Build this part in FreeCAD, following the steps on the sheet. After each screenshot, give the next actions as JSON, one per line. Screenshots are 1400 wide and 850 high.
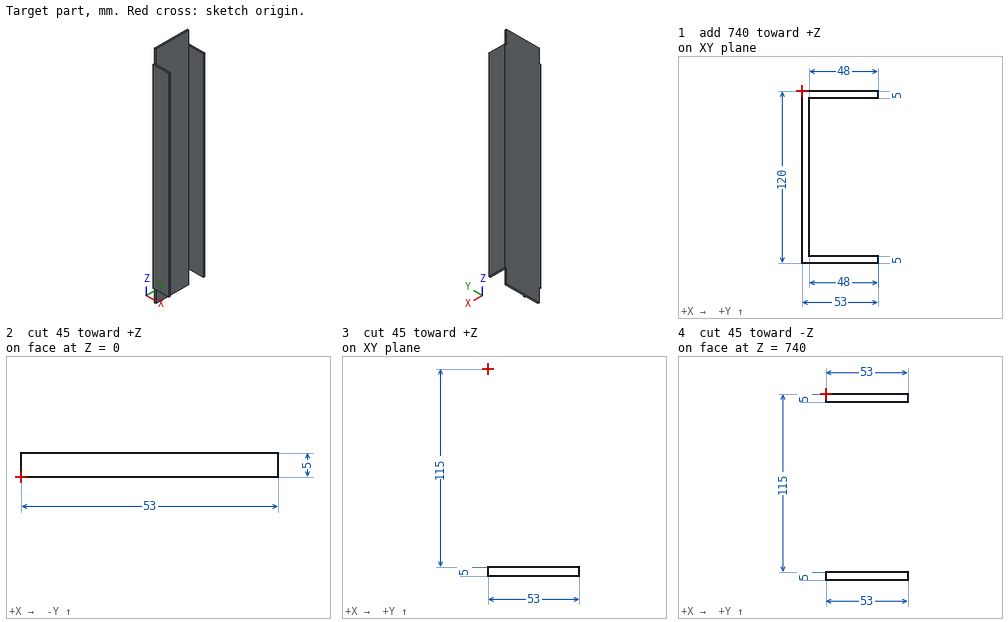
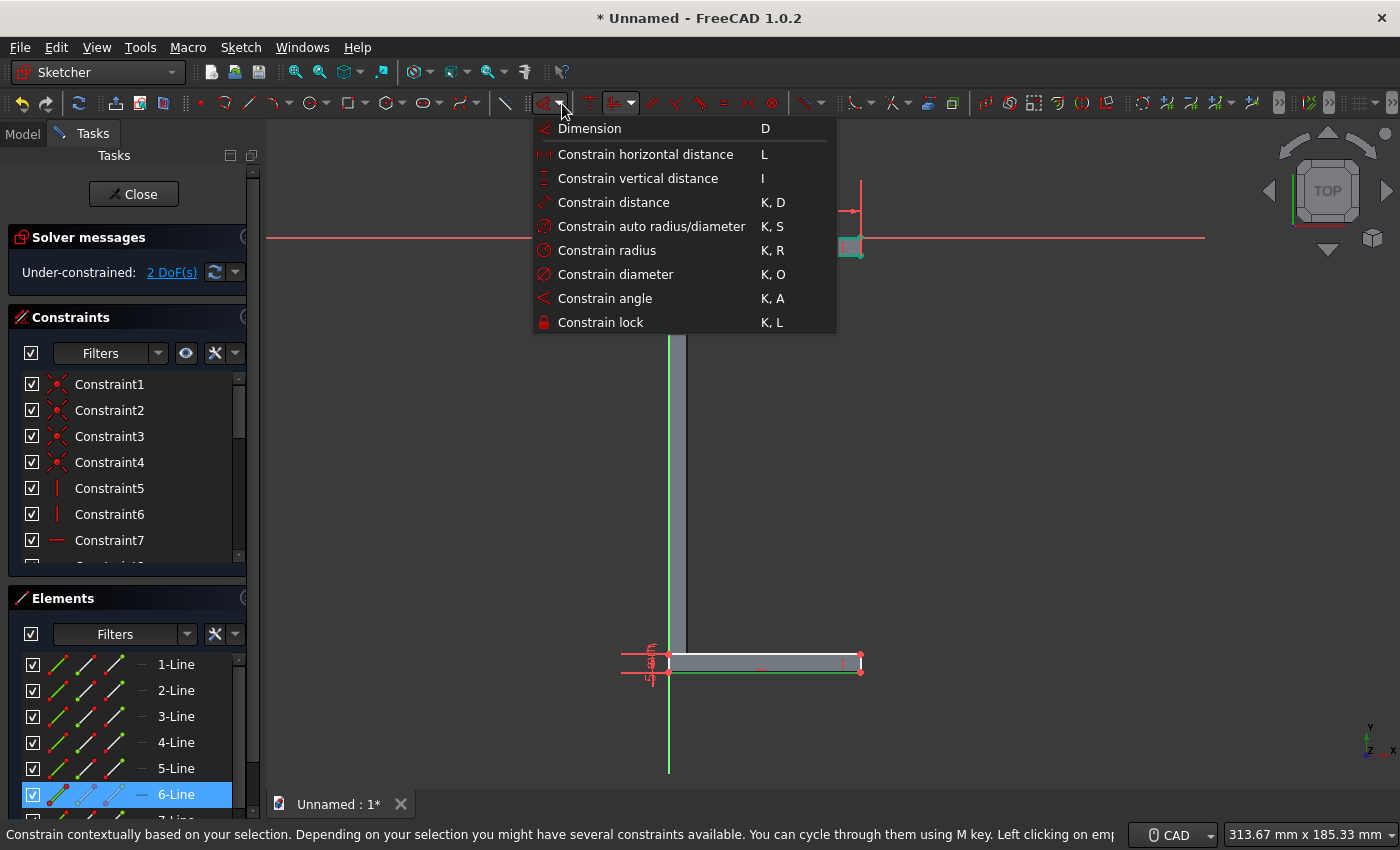
{"action": "left_click", "coordinate": [685, 154]}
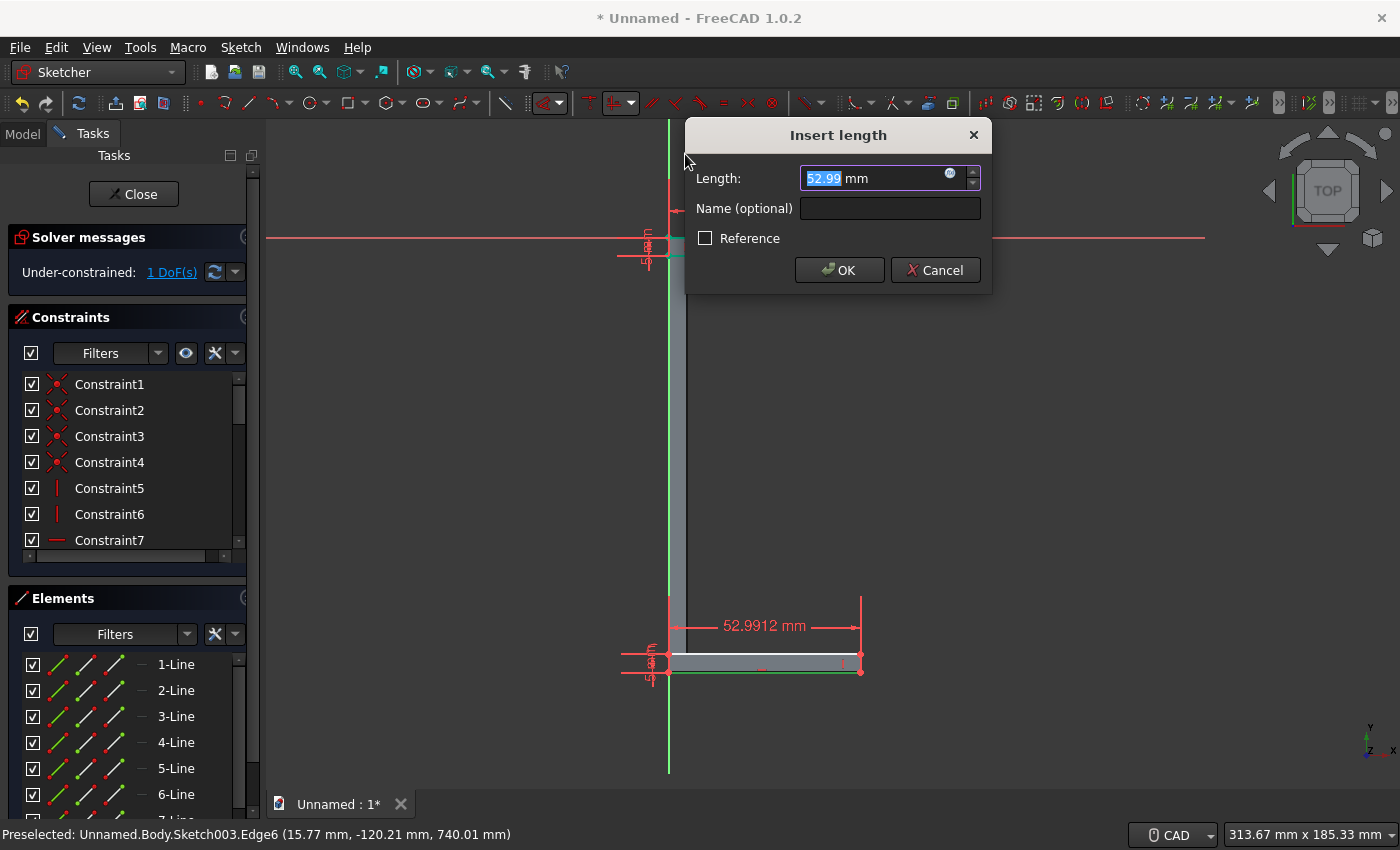
{"action": "type", "text": "53"}
{"action": "key", "text": "Return"}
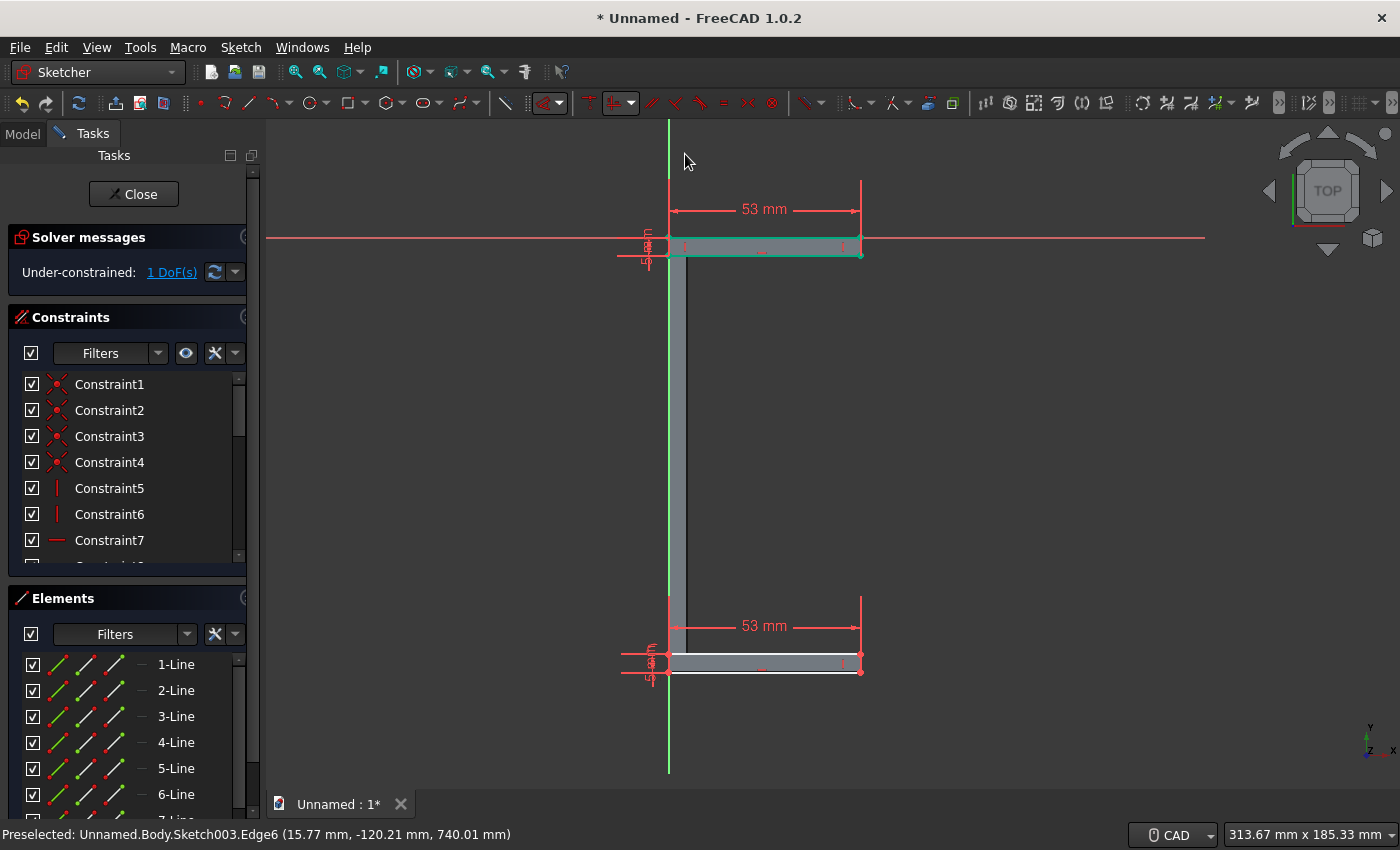
{"action": "left_click", "coordinate": [669, 654]}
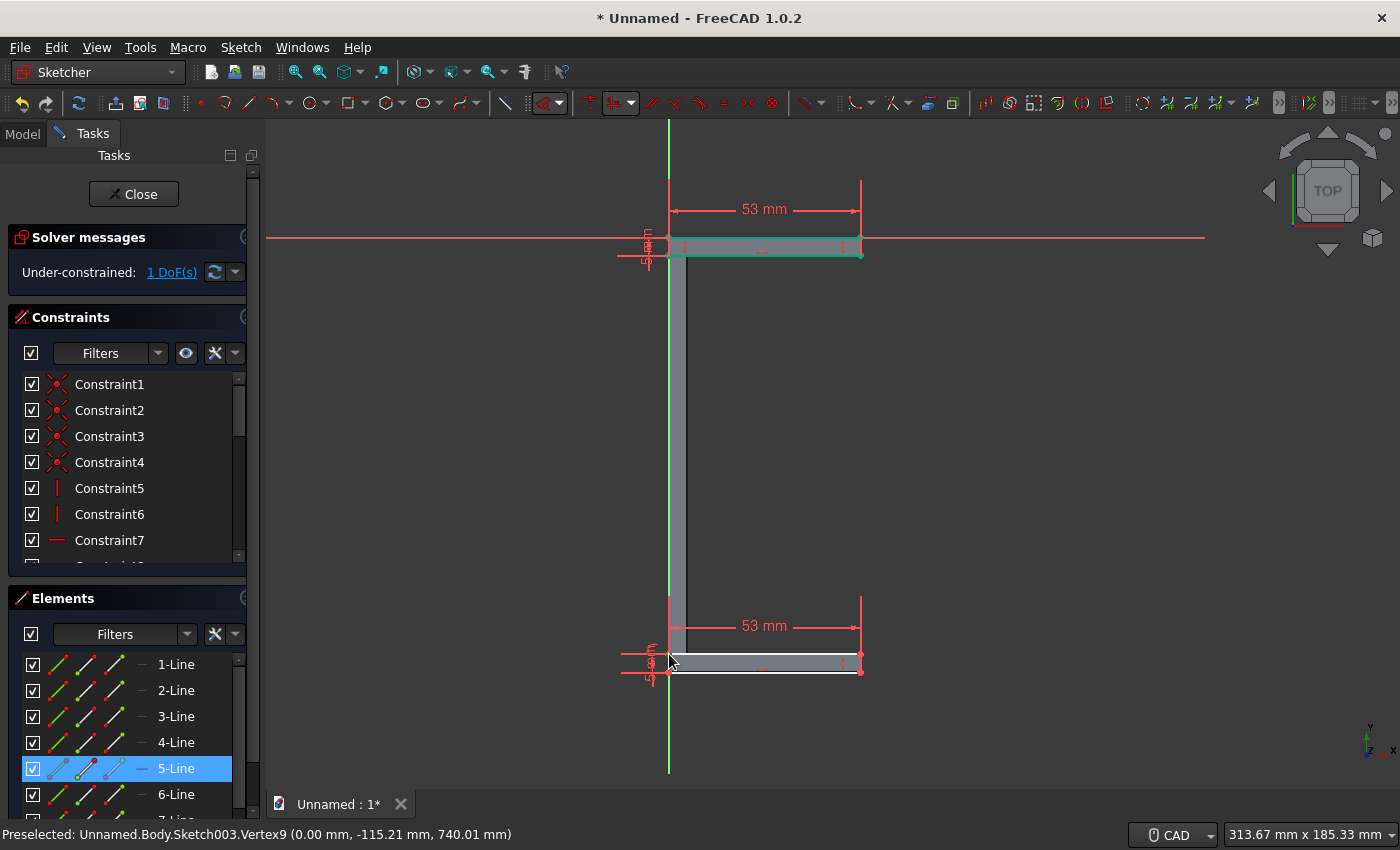
{"action": "left_click", "coordinate": [562, 104]}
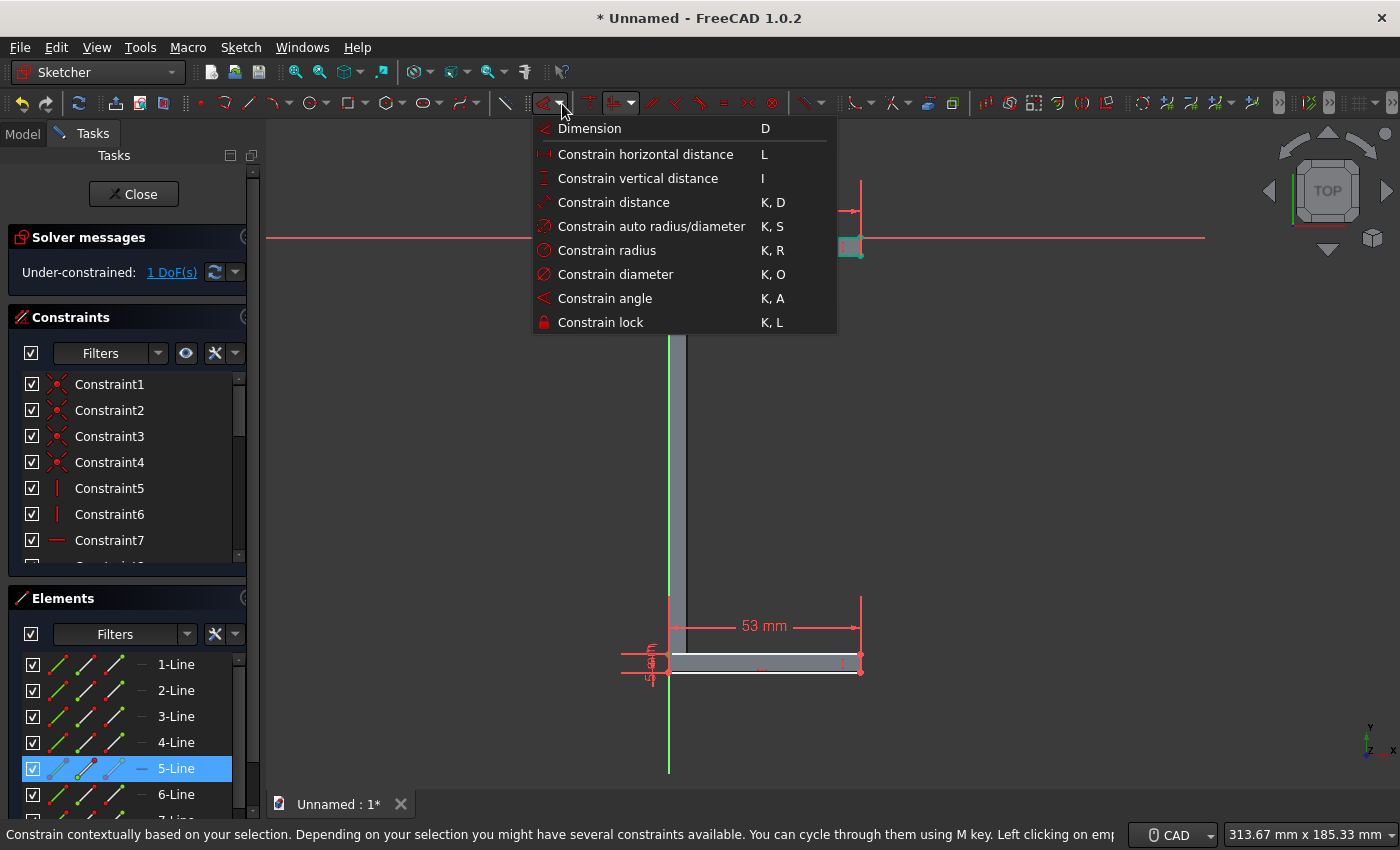
{"action": "left_click", "coordinate": [685, 178]}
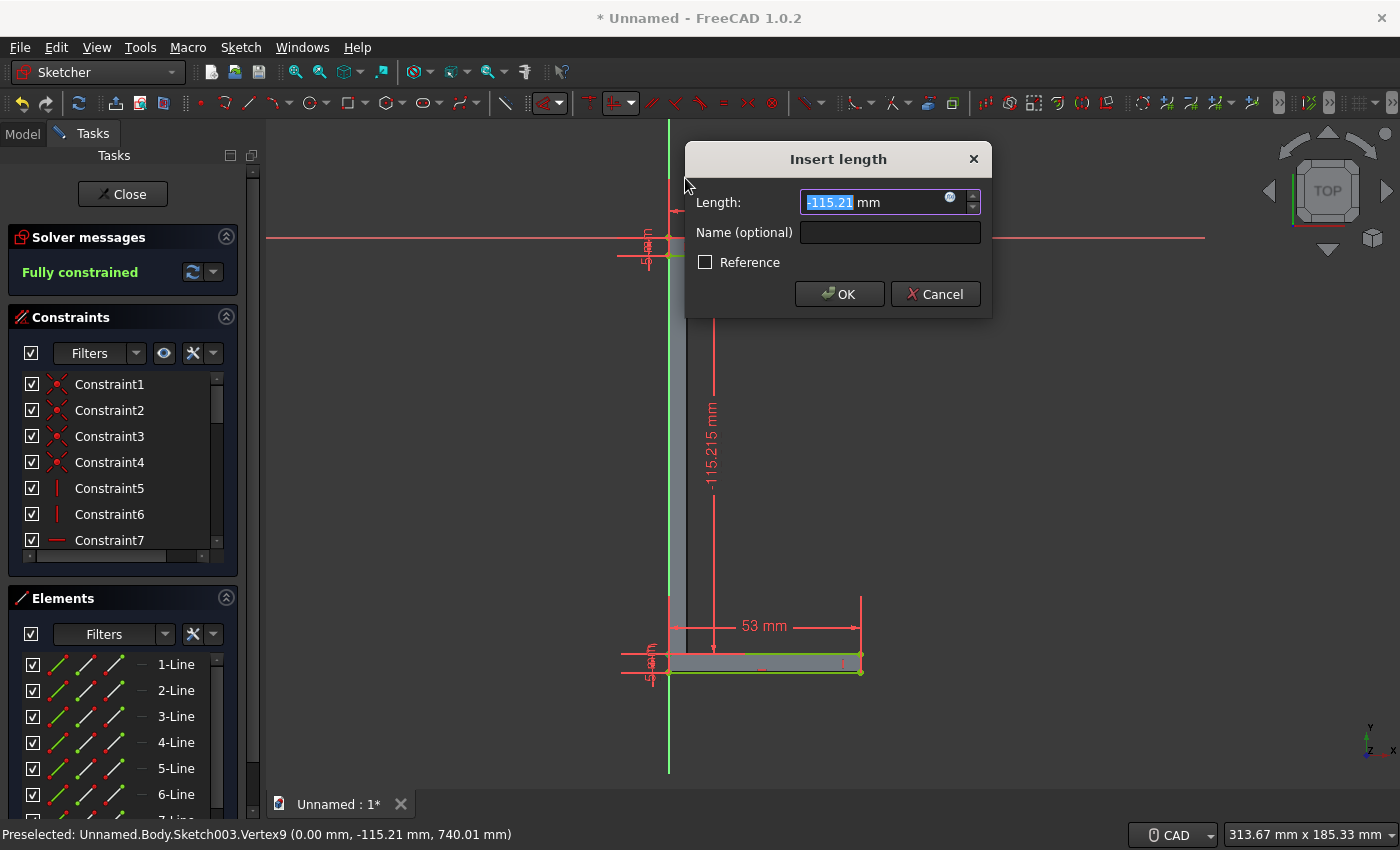
{"action": "type", "text": "-115"}
{"action": "key", "text": "Return"}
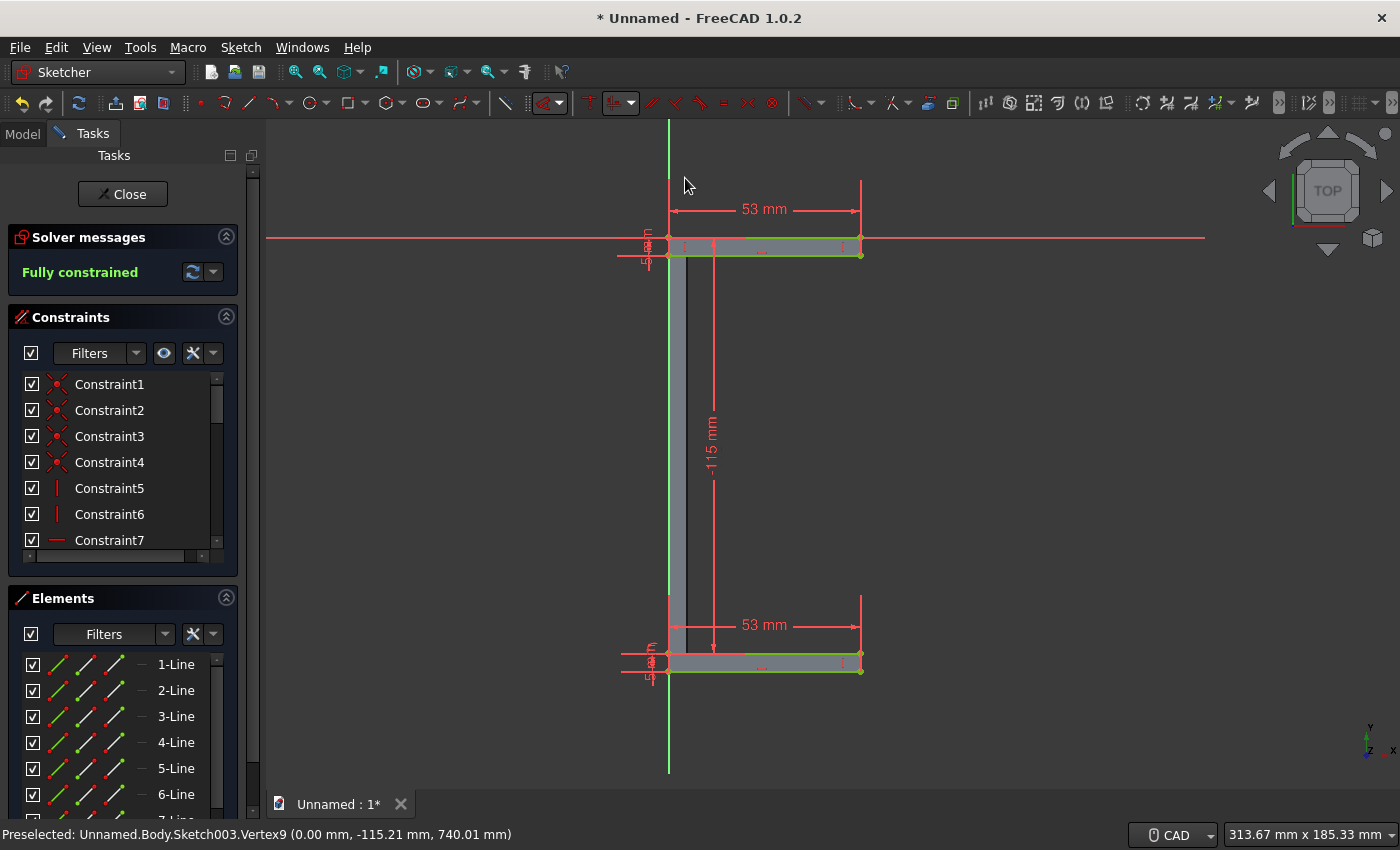
{"action": "left_click", "coordinate": [123, 194]}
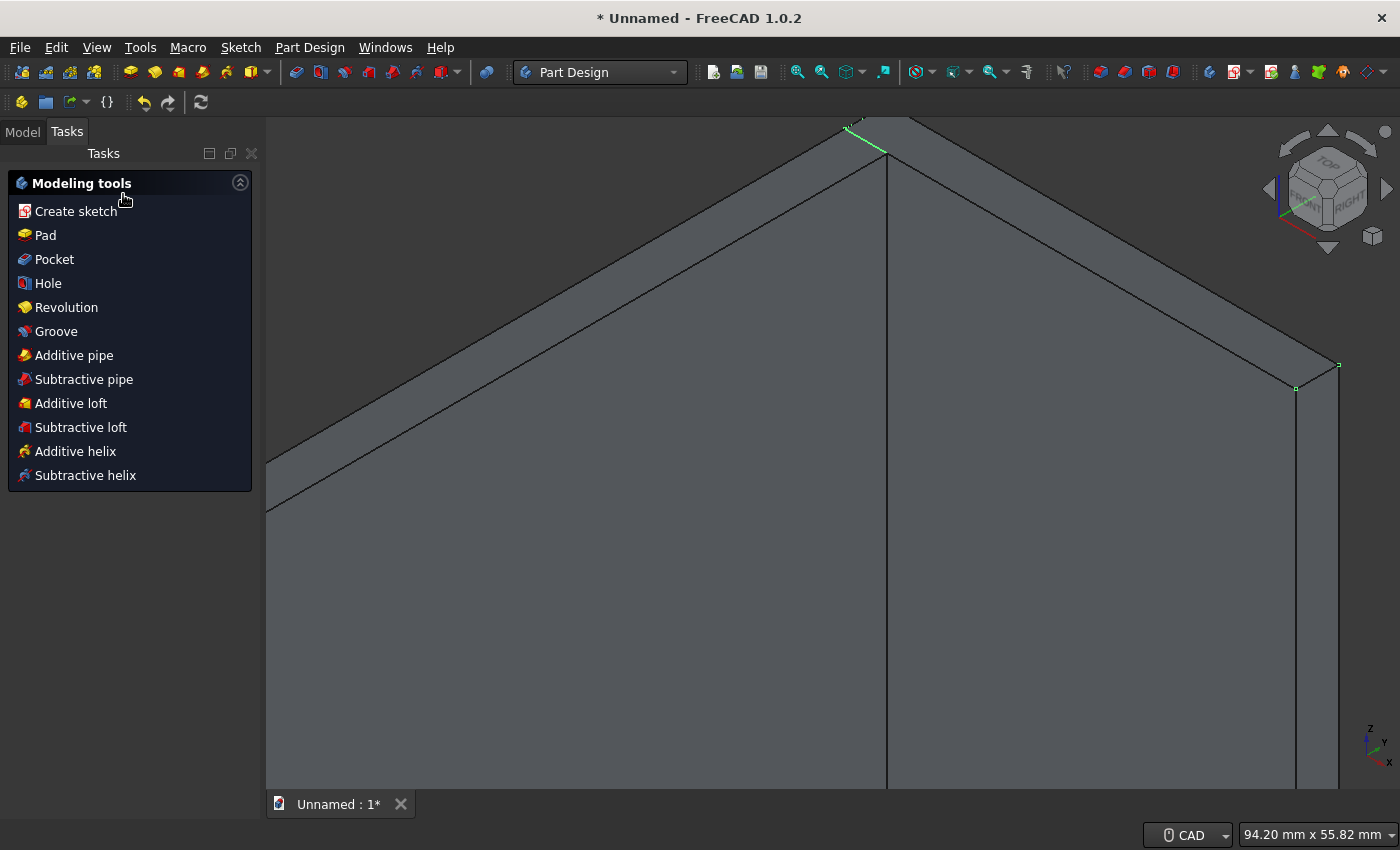
{"action": "left_click", "coordinate": [298, 72]}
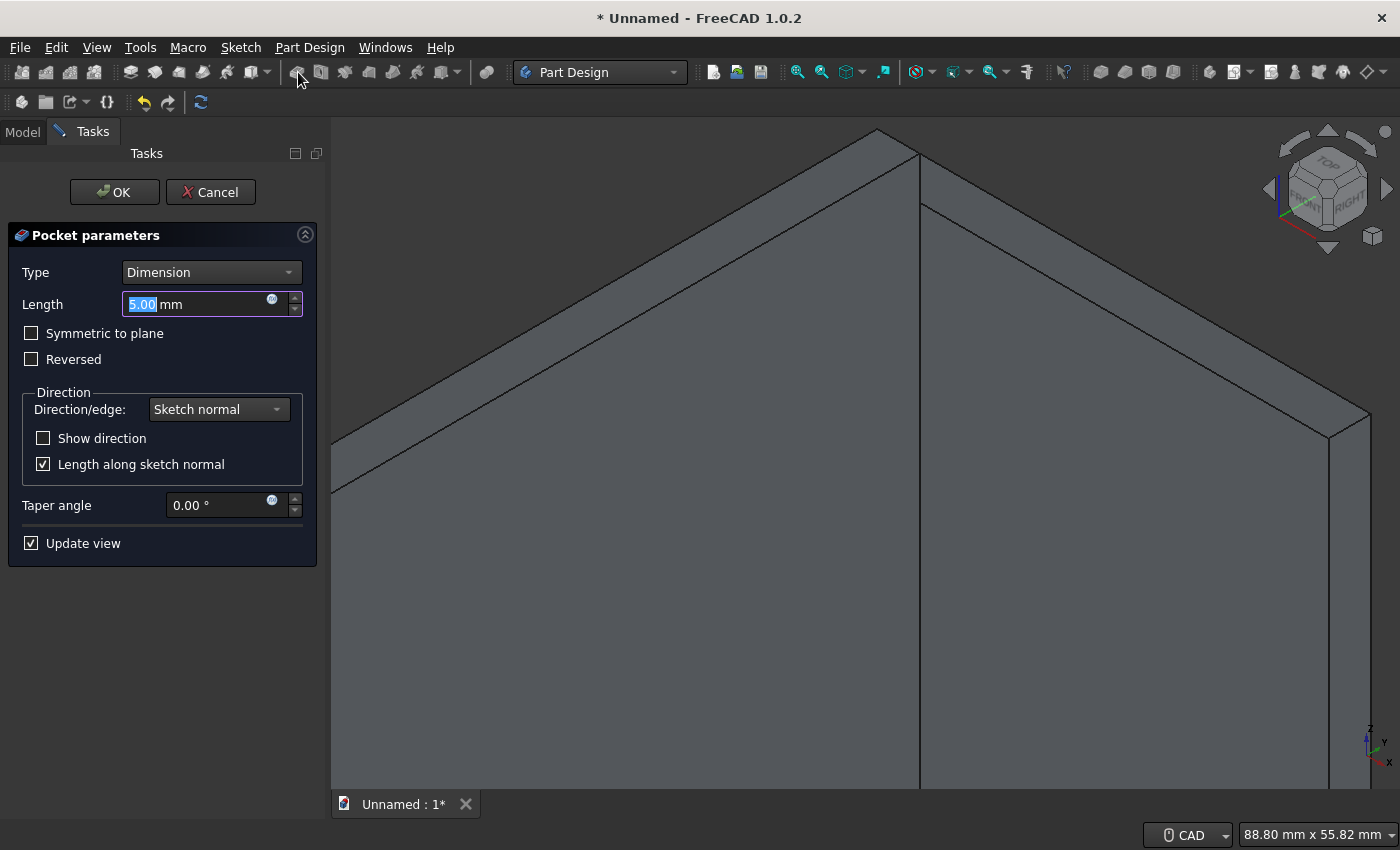
{"action": "type", "text": "45"}
{"action": "key", "text": "Tab"}